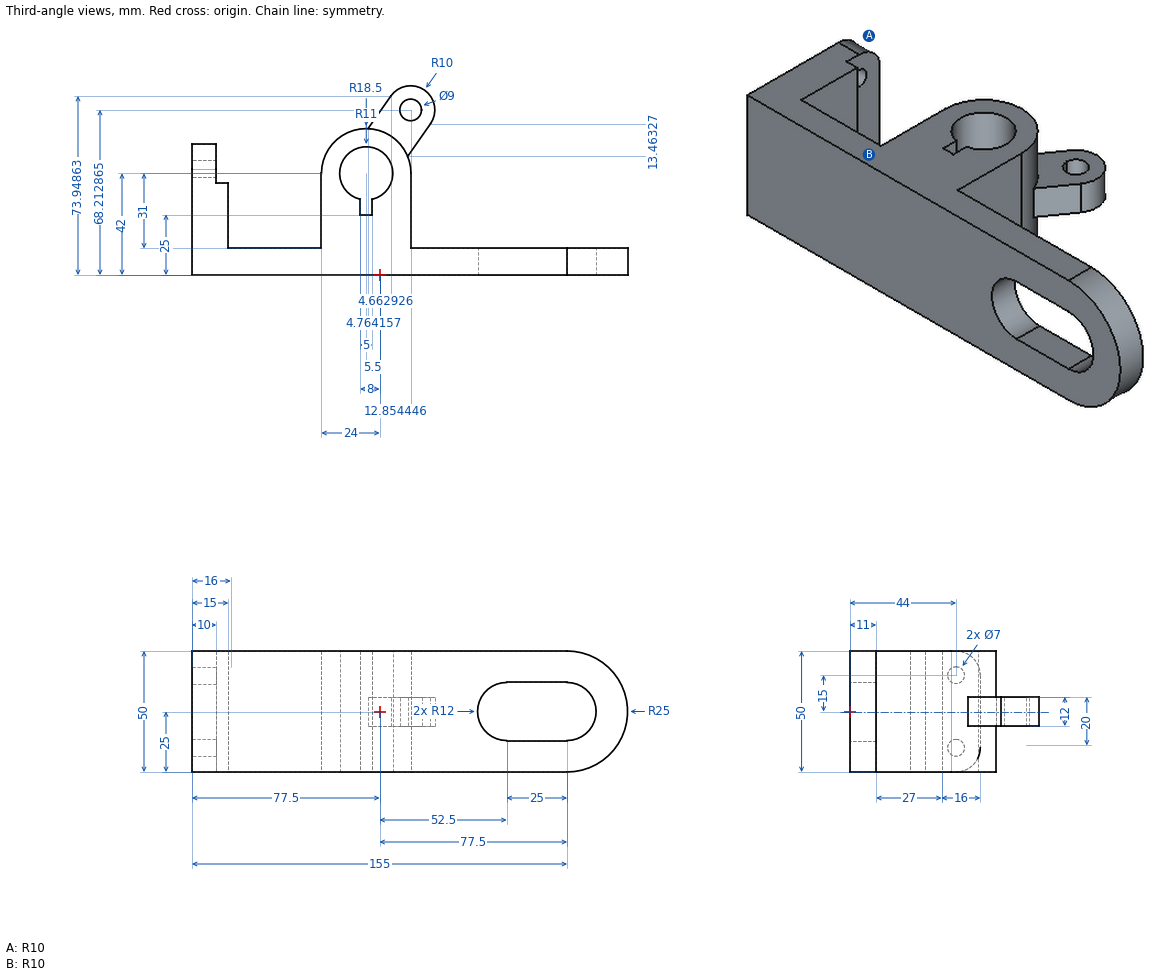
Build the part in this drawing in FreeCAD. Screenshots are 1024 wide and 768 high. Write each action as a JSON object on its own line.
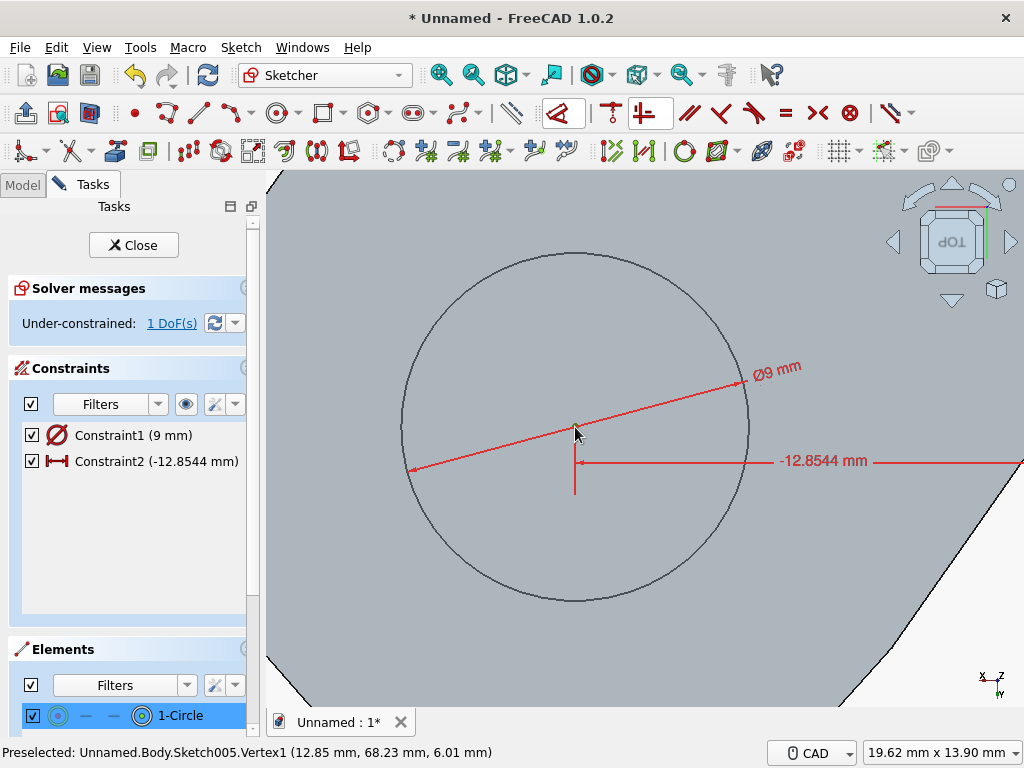
{"action": "left_click", "coordinate": [580, 114]}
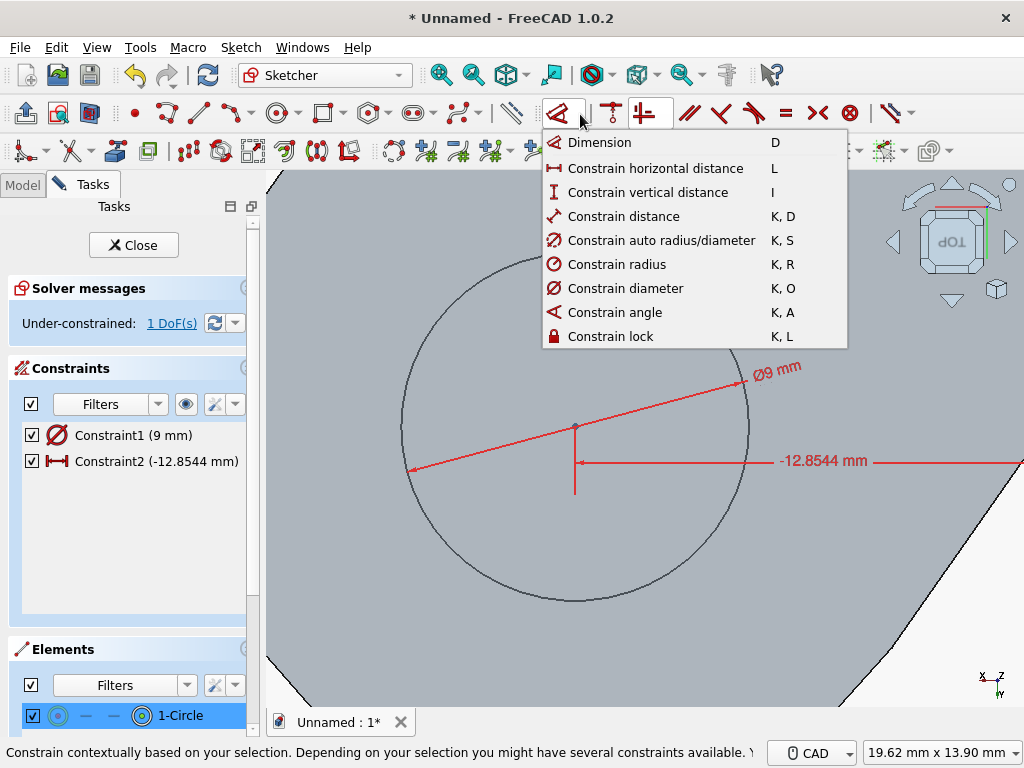
{"action": "left_click", "coordinate": [695, 192]}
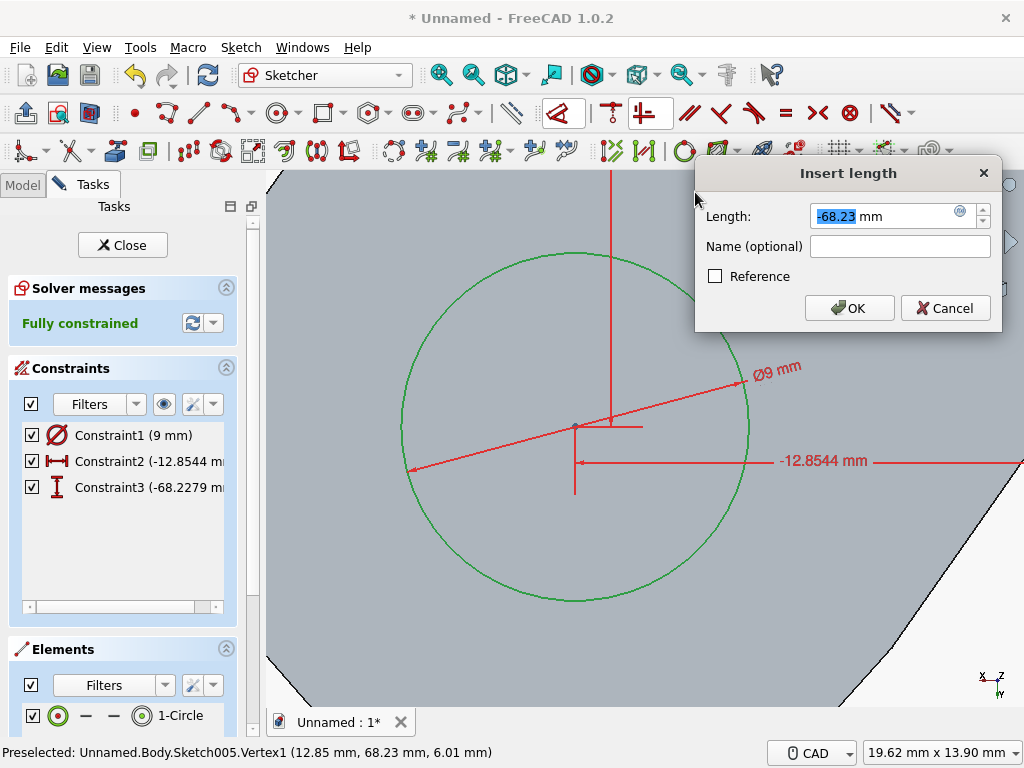
{"action": "type", "text": "-68.212865"}
{"action": "key", "text": "Return"}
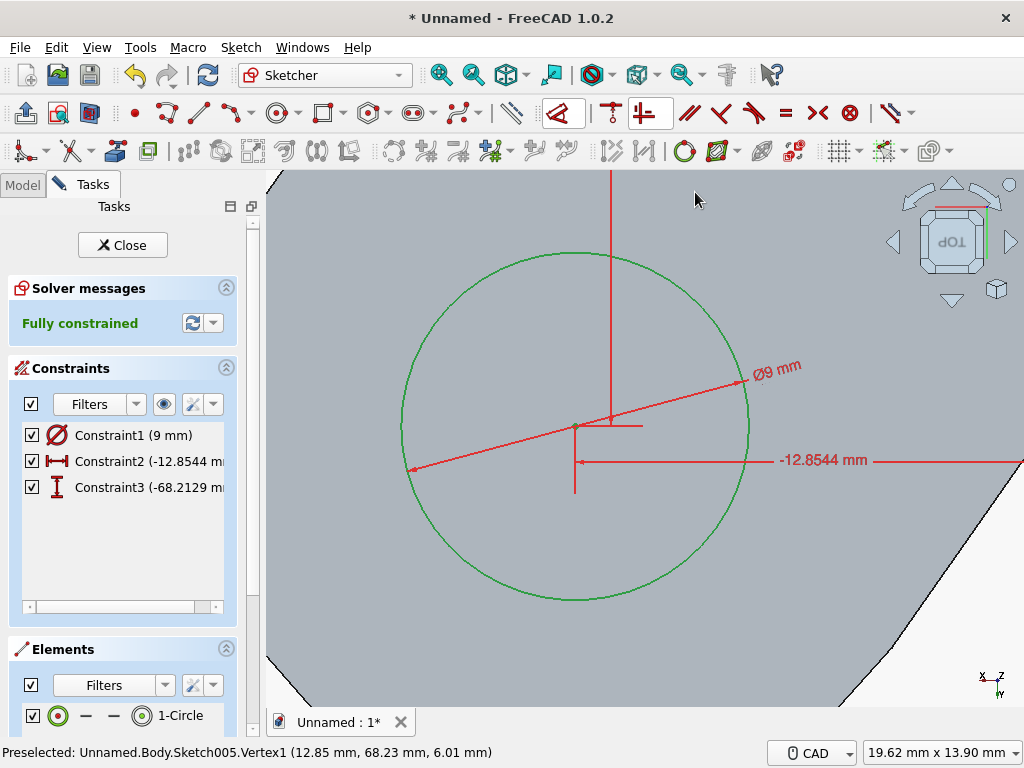
{"action": "left_click", "coordinate": [123, 245]}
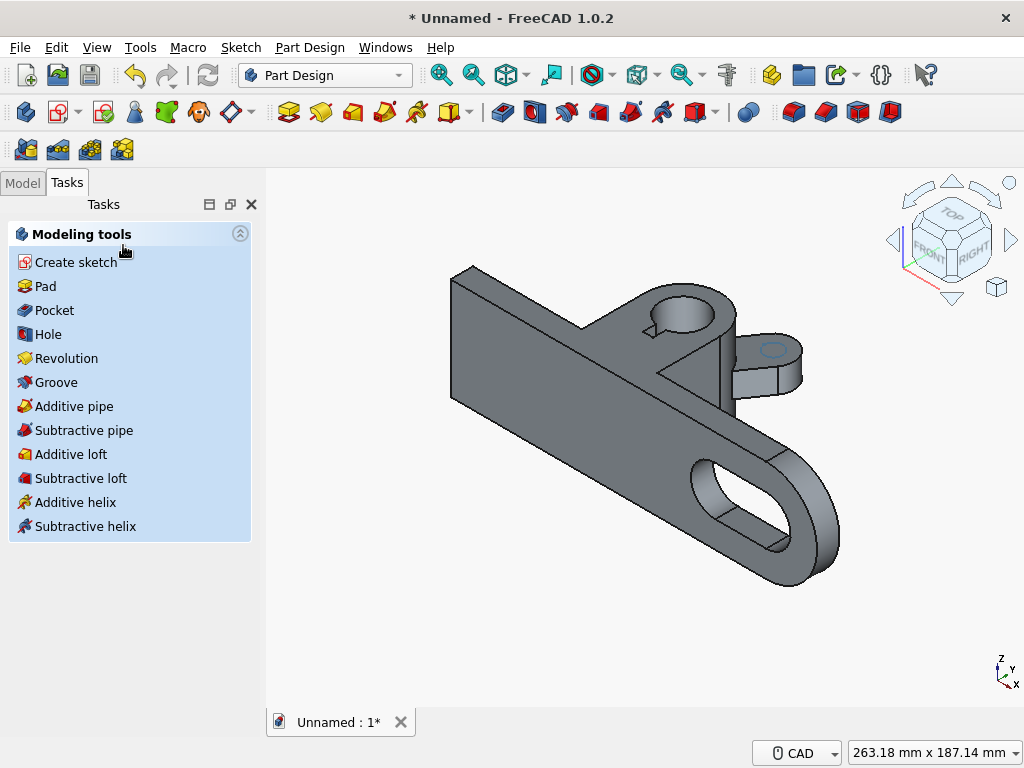
{"action": "left_click", "coordinate": [504, 112]}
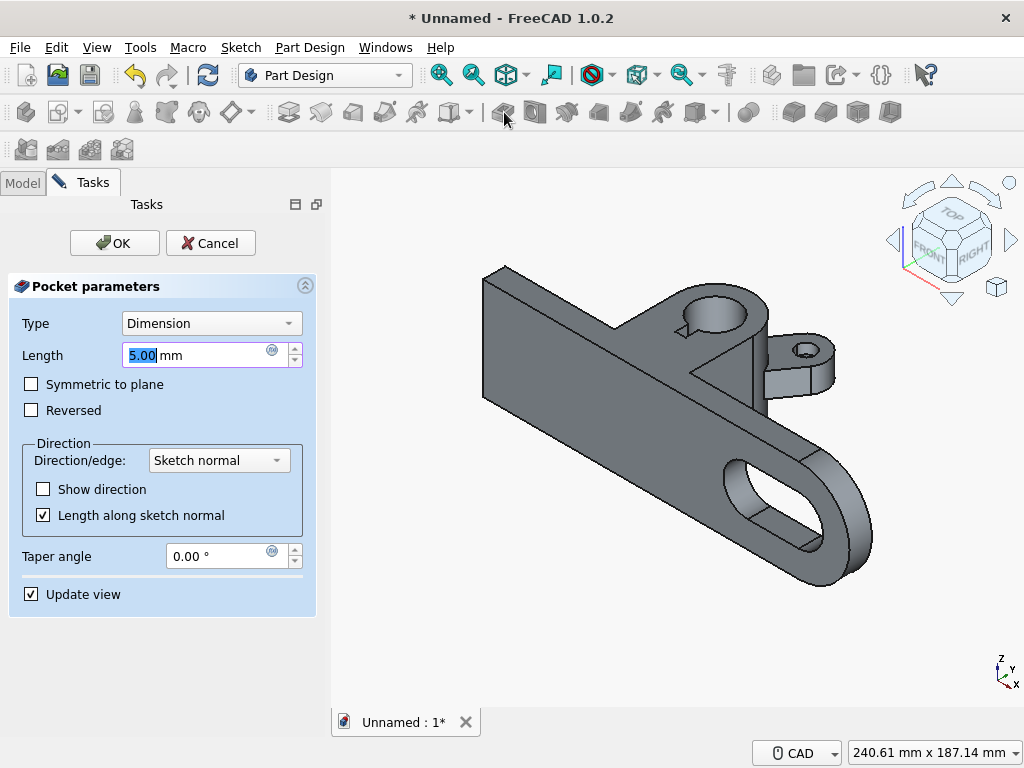
{"action": "type", "text": "20"}
{"action": "key", "text": "Tab"}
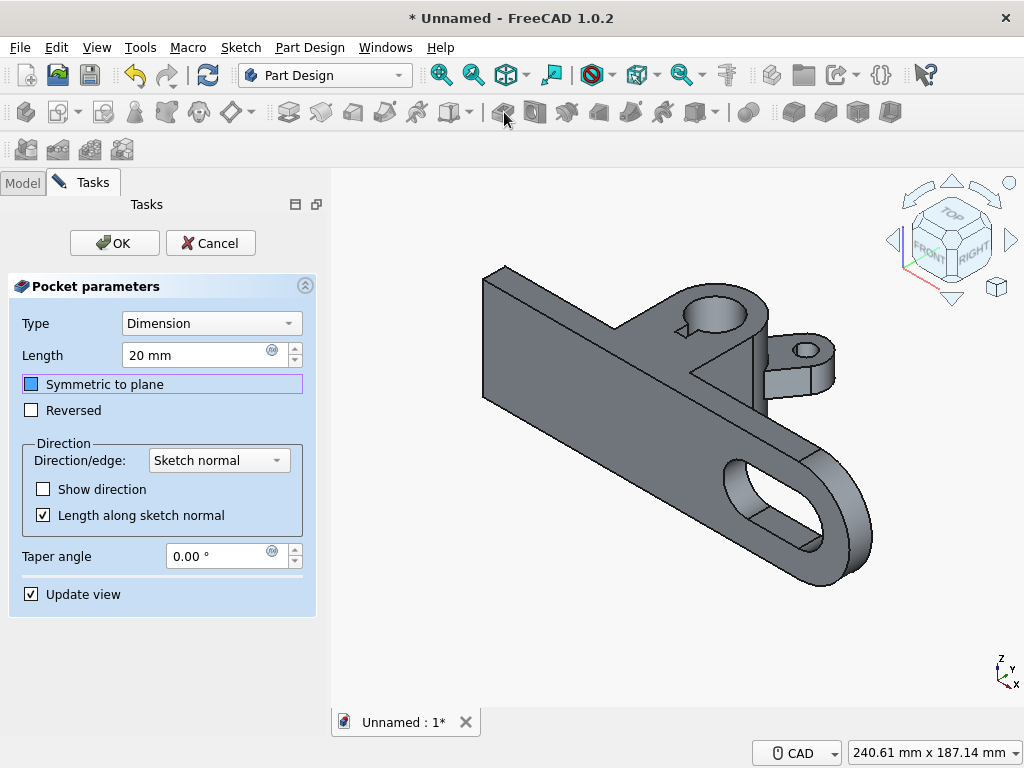
{"action": "left_click", "coordinate": [115, 243]}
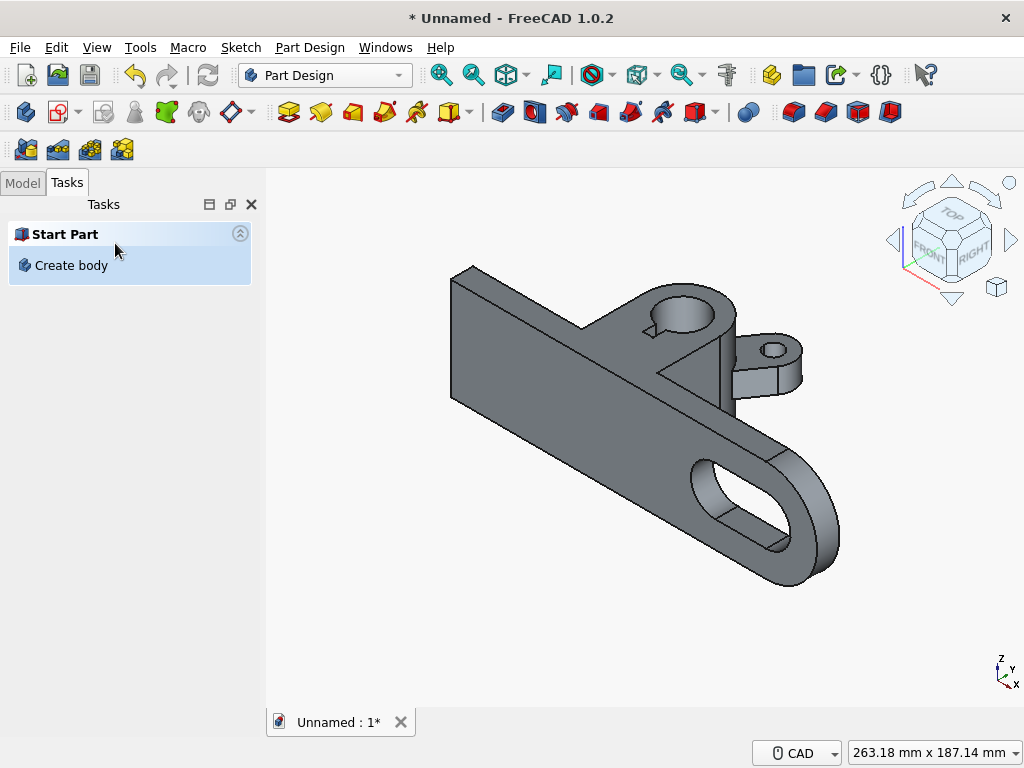
{"action": "key", "text": "4"}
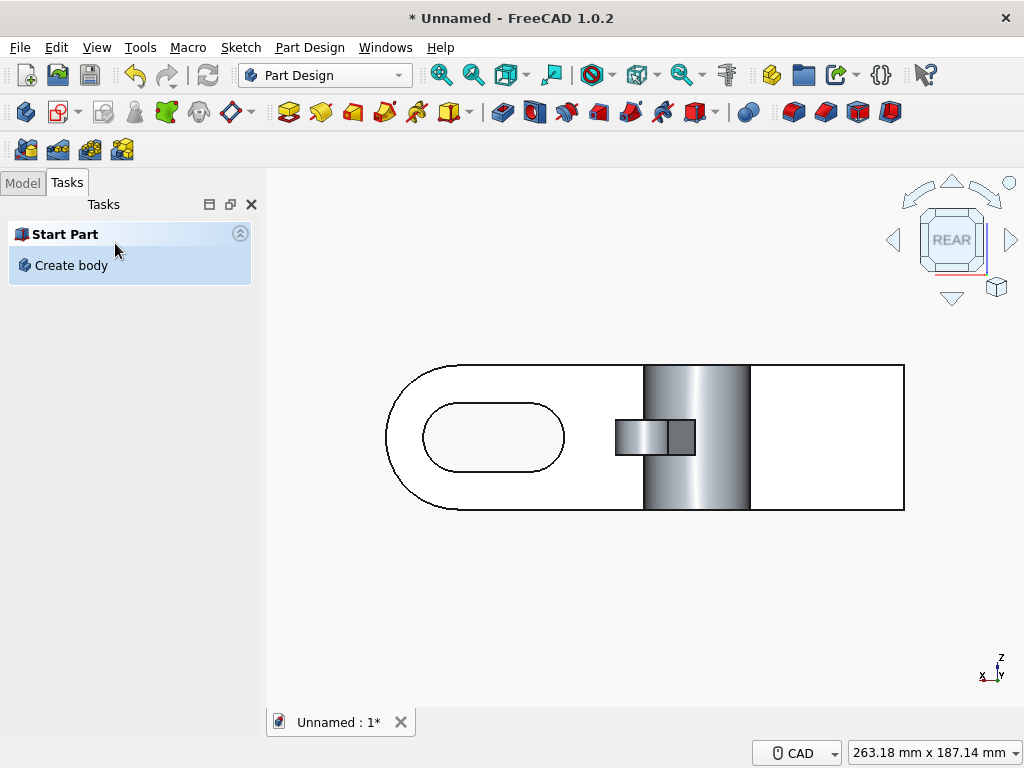
{"action": "left_click", "coordinate": [588, 478]}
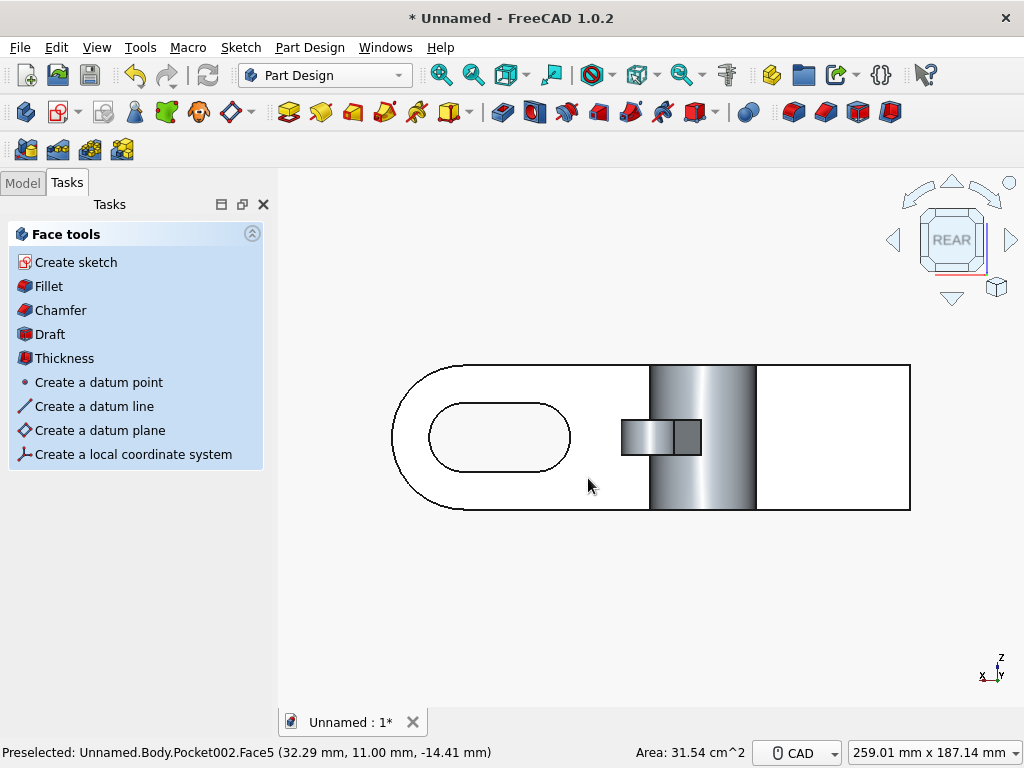
{"action": "left_click", "coordinate": [58, 112]}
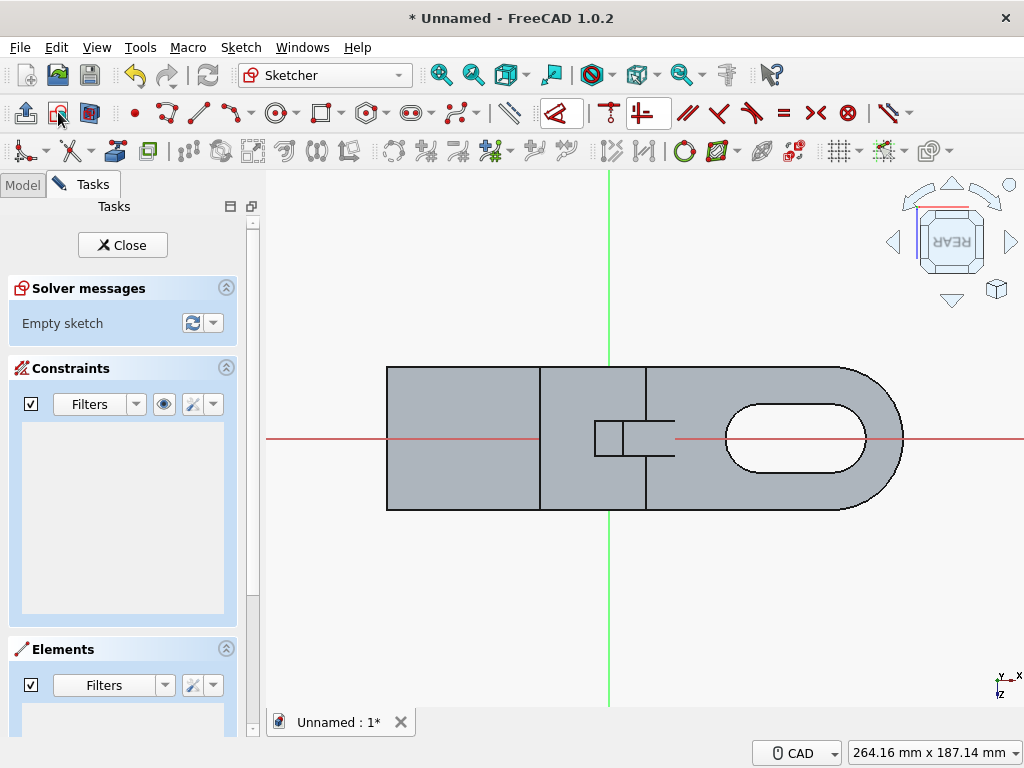
{"action": "left_click", "coordinate": [90, 114]}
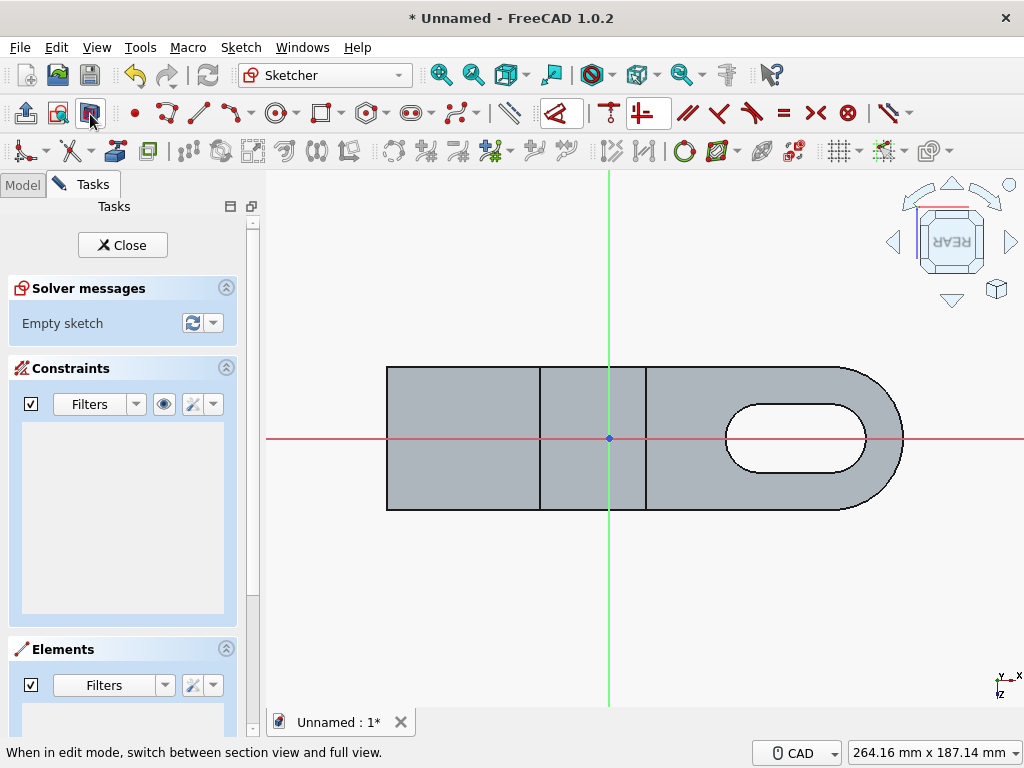
{"action": "scroll", "coordinate": [402, 438], "scroll_direction": "up", "scroll_amount": 3}